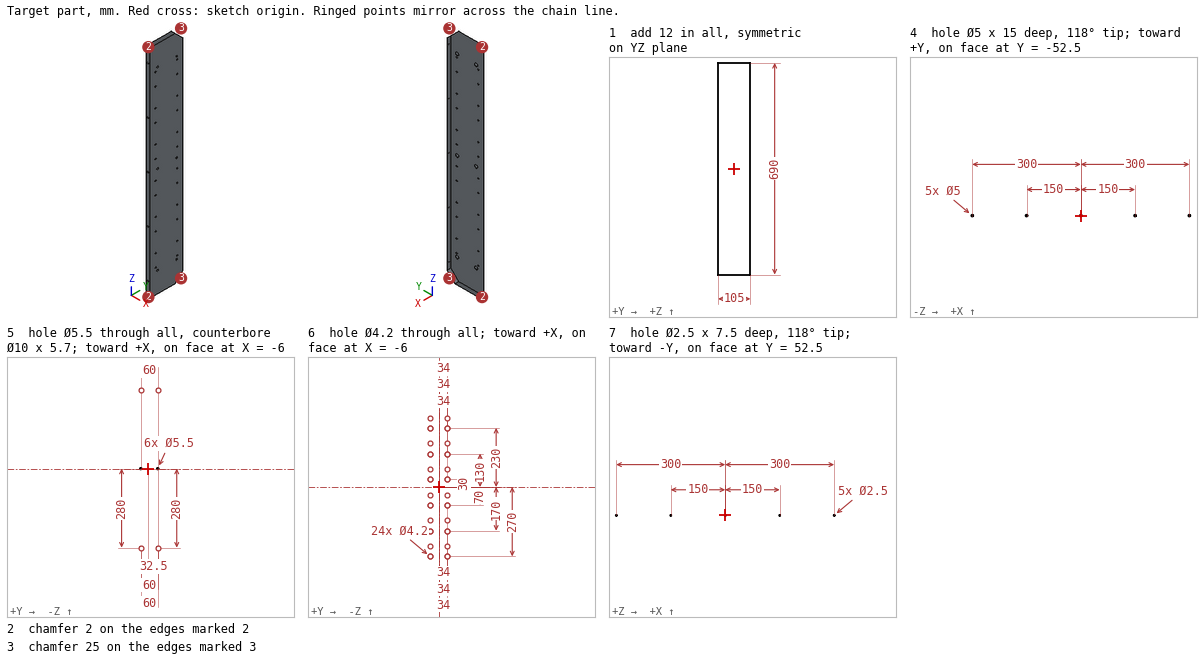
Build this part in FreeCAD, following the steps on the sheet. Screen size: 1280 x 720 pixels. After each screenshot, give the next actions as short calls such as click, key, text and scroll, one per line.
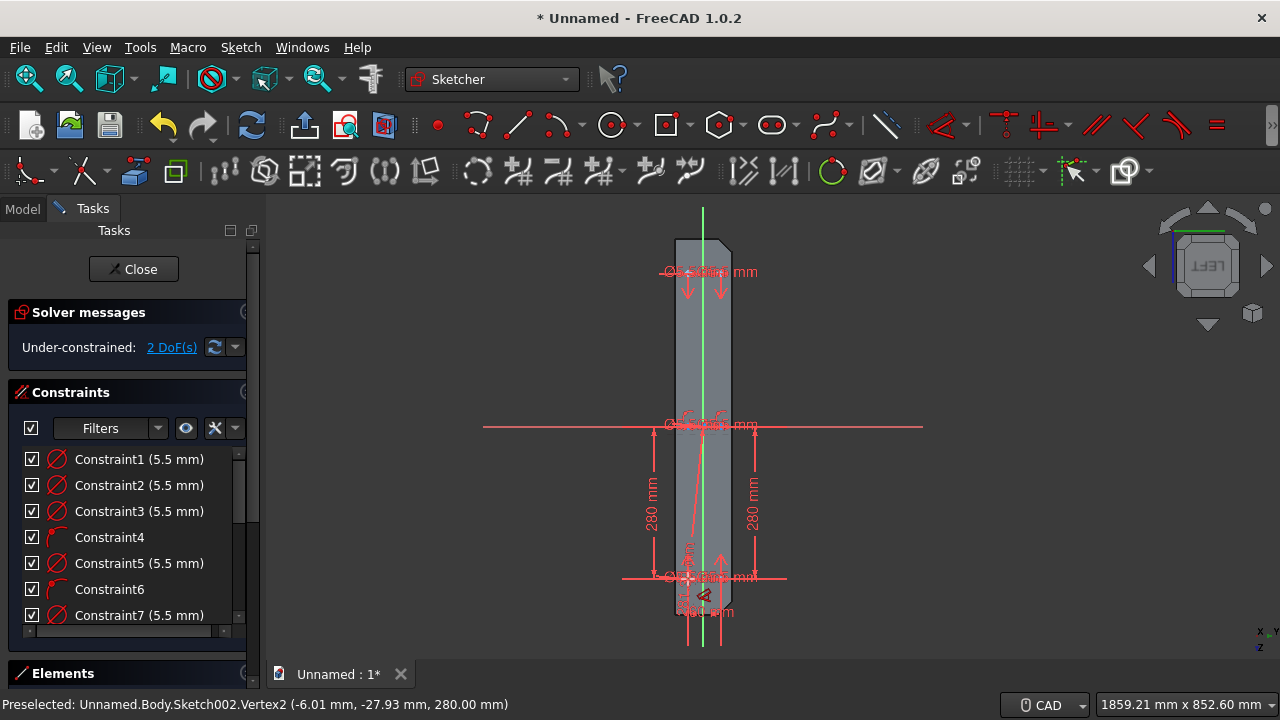
click(721, 427)
click(712, 393)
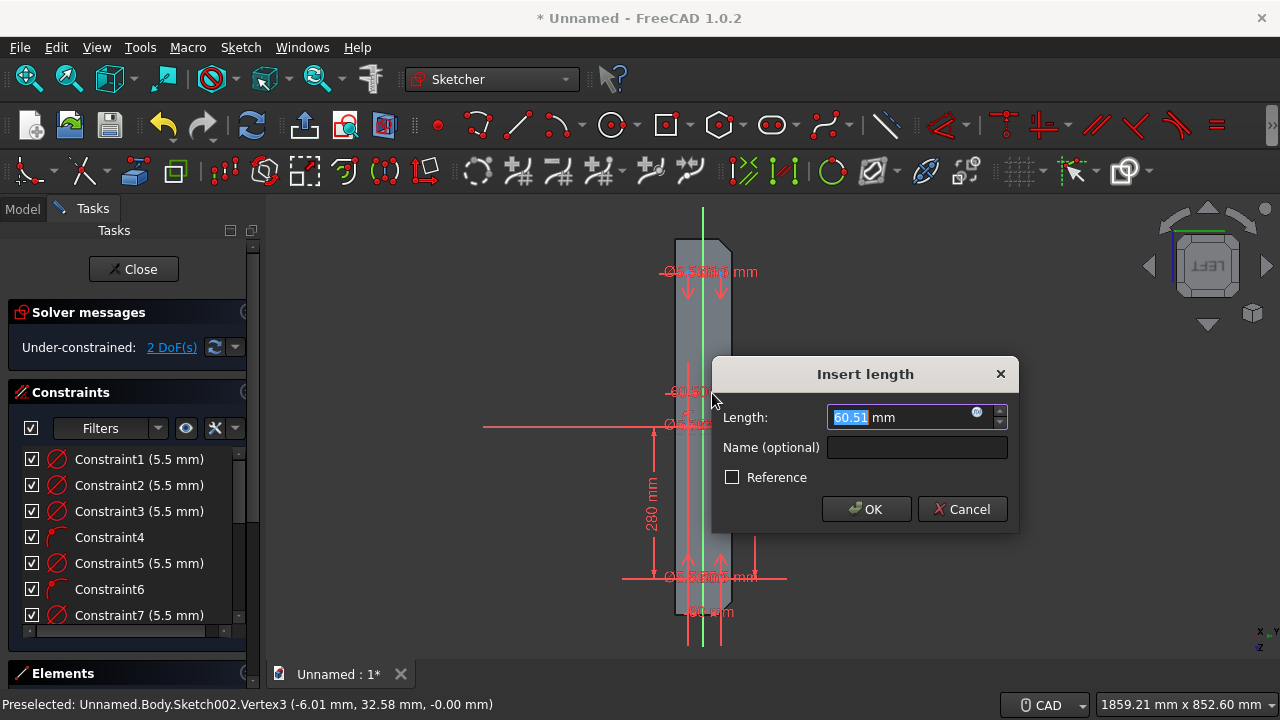
text(60)
key(Return)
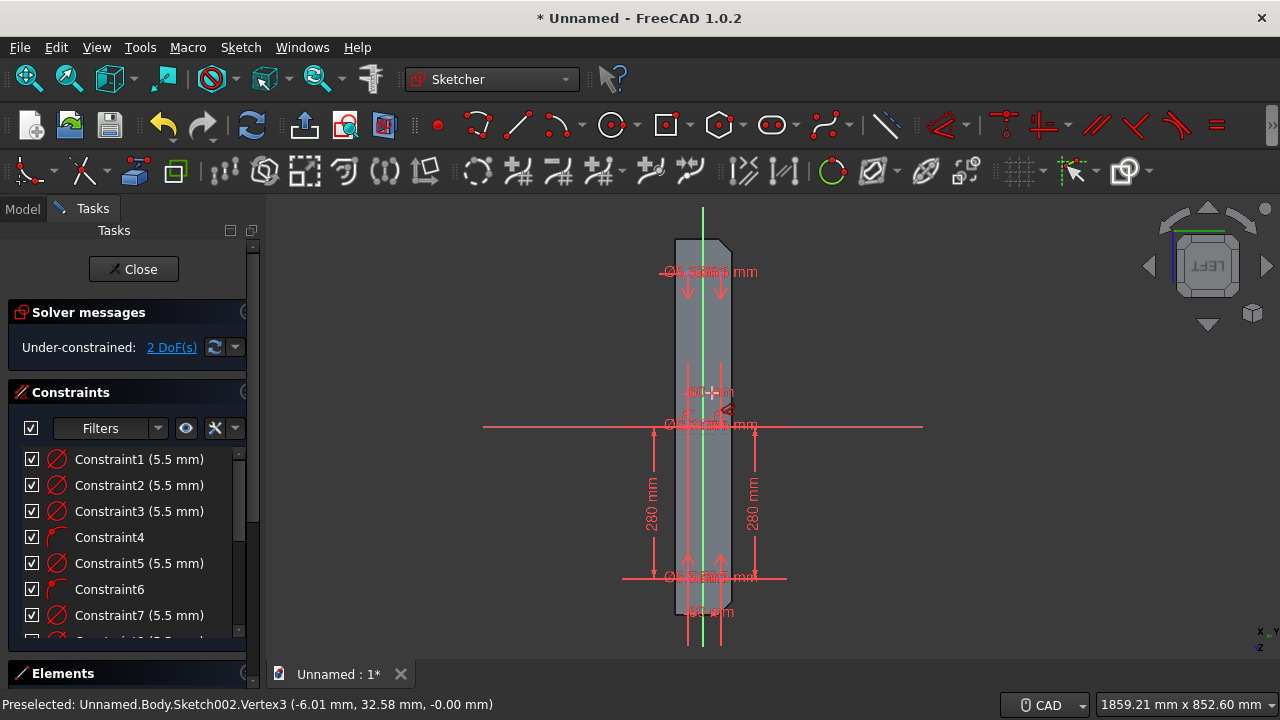
click(721, 427)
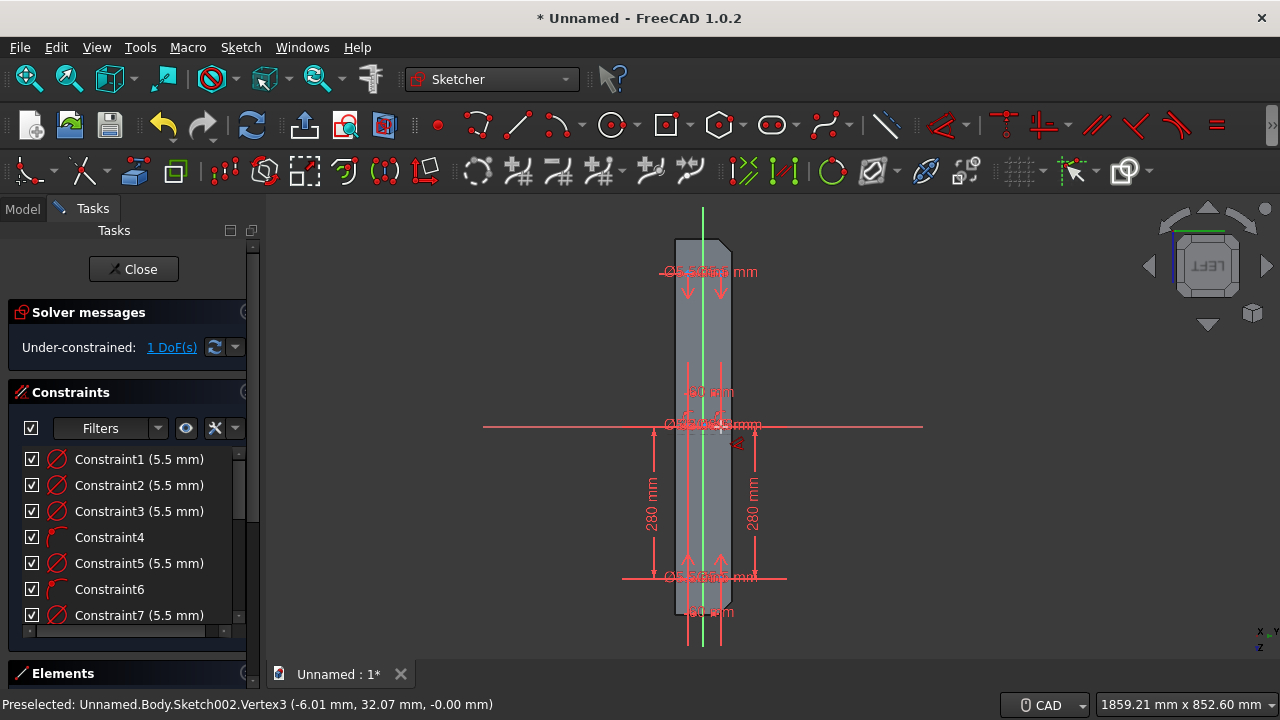
click(688, 427)
click(712, 461)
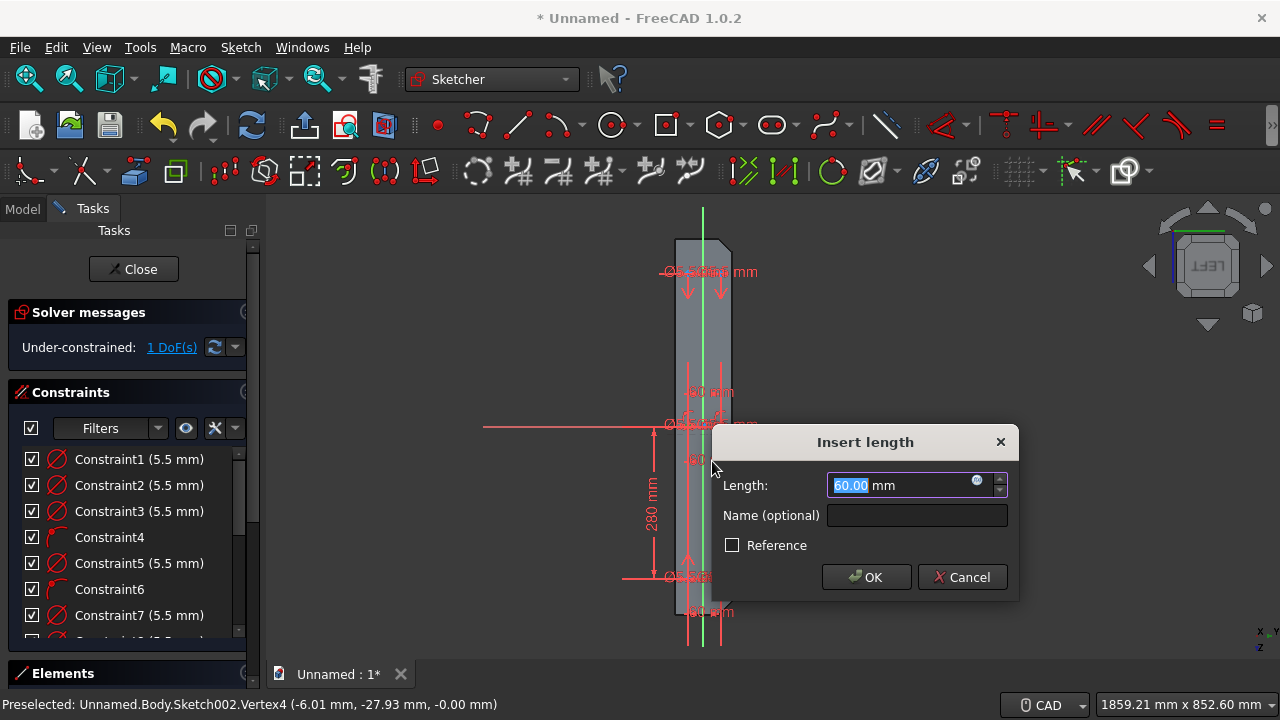
text(60)
key(Return)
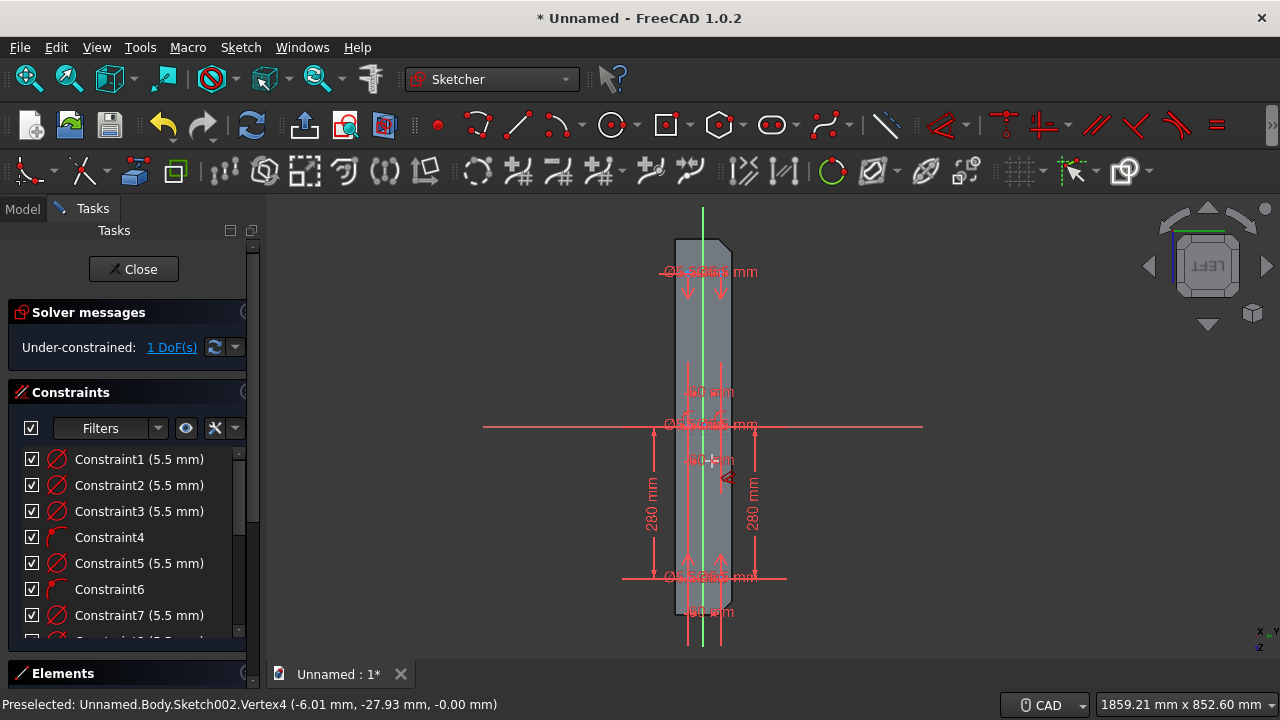
scroll(721, 579, up, 5)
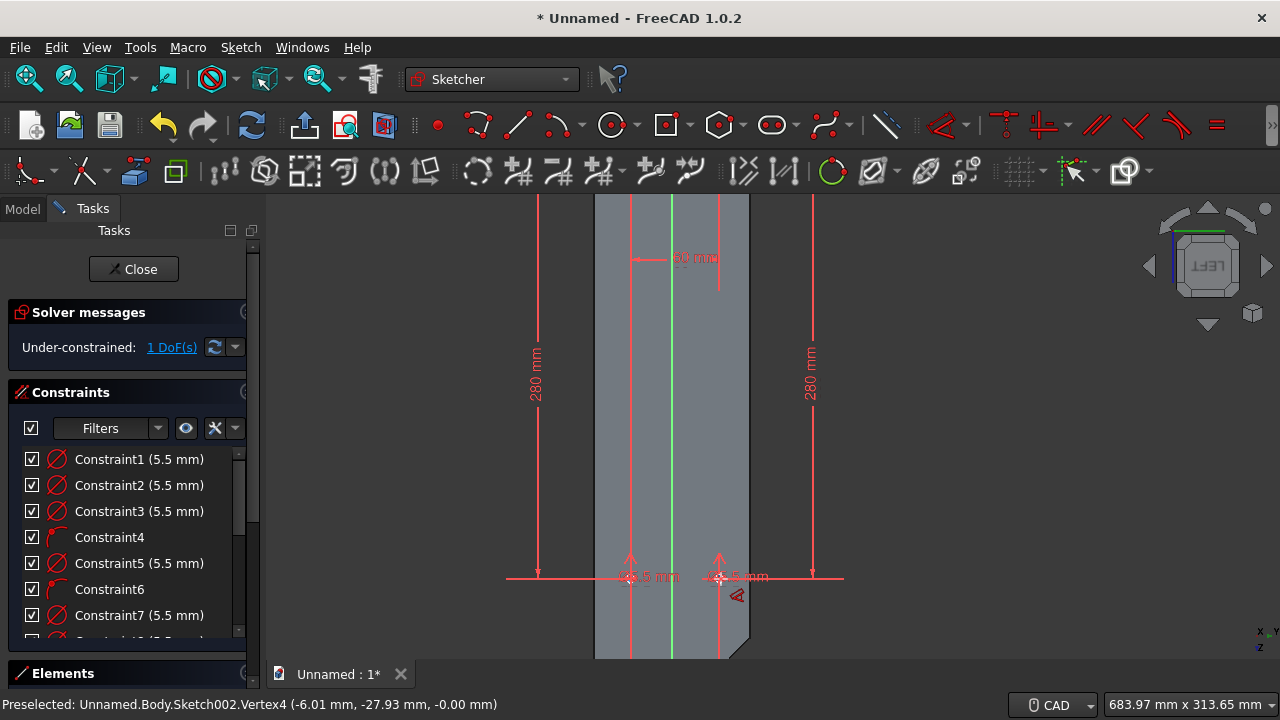
click(719, 579)
click(696, 613)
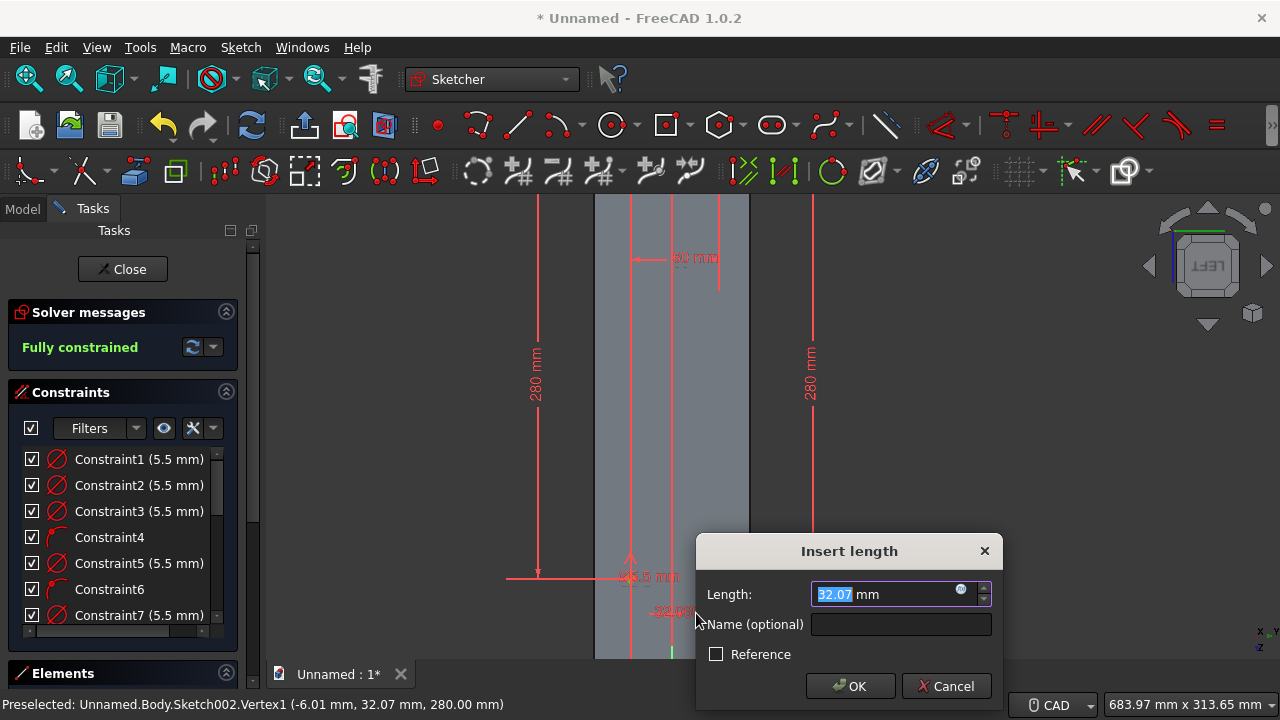
text(32.5)
key(Return)
key(Escape)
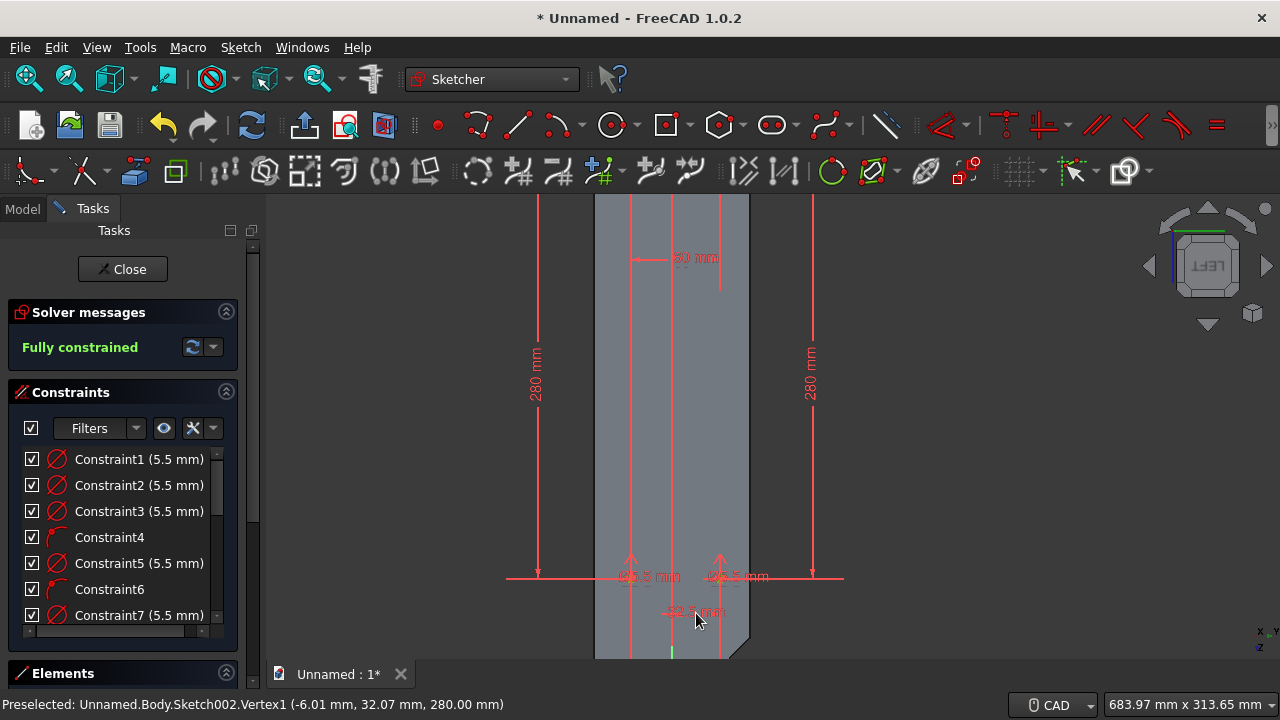
click(123, 269)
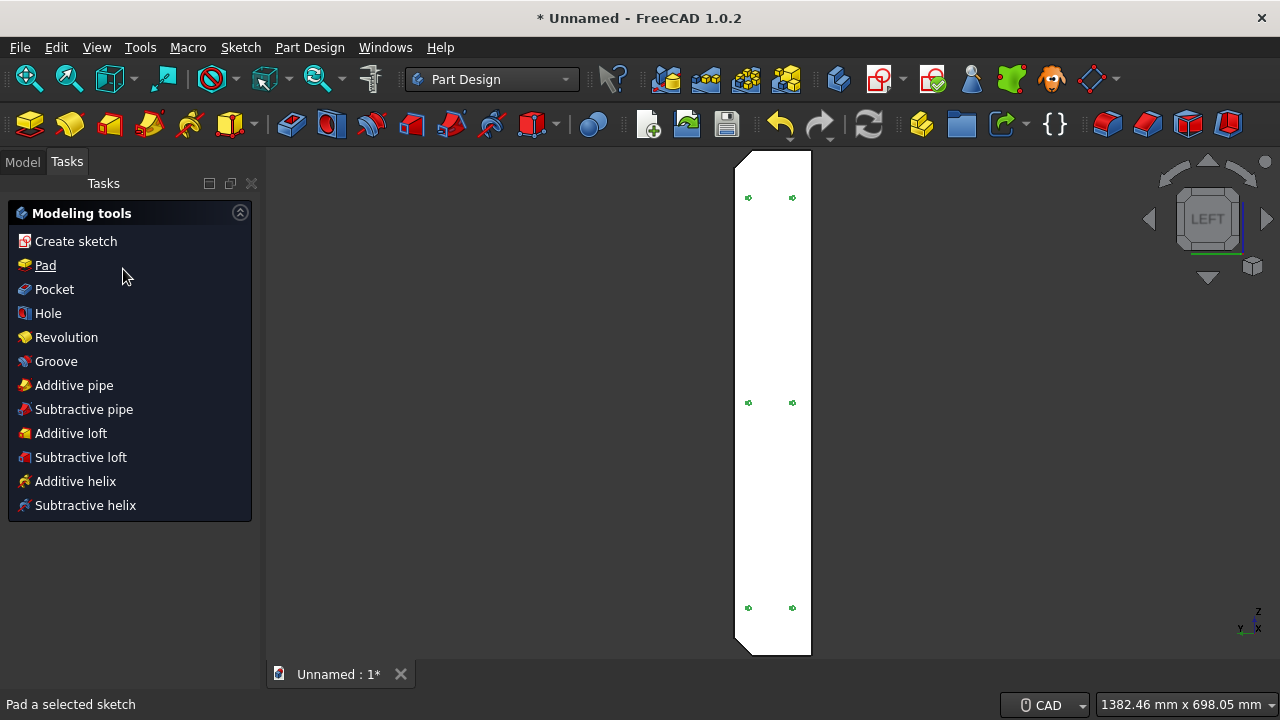
click(332, 124)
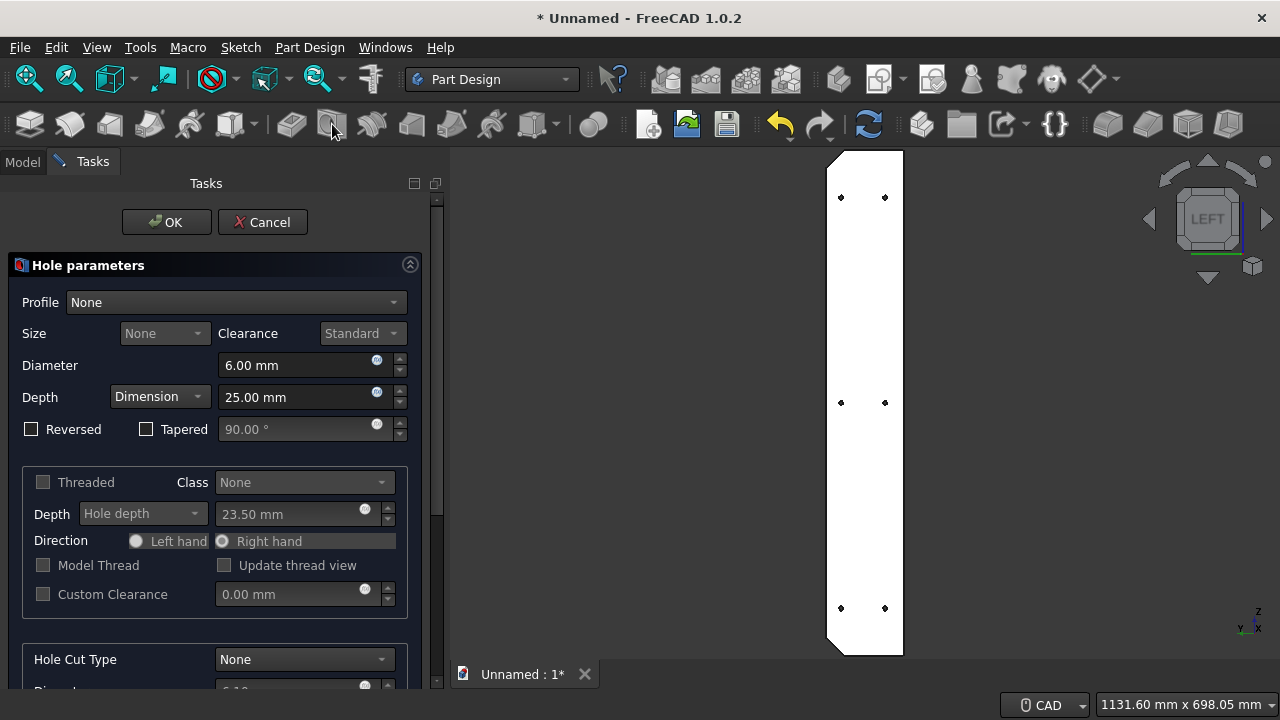
triple_click(305, 365)